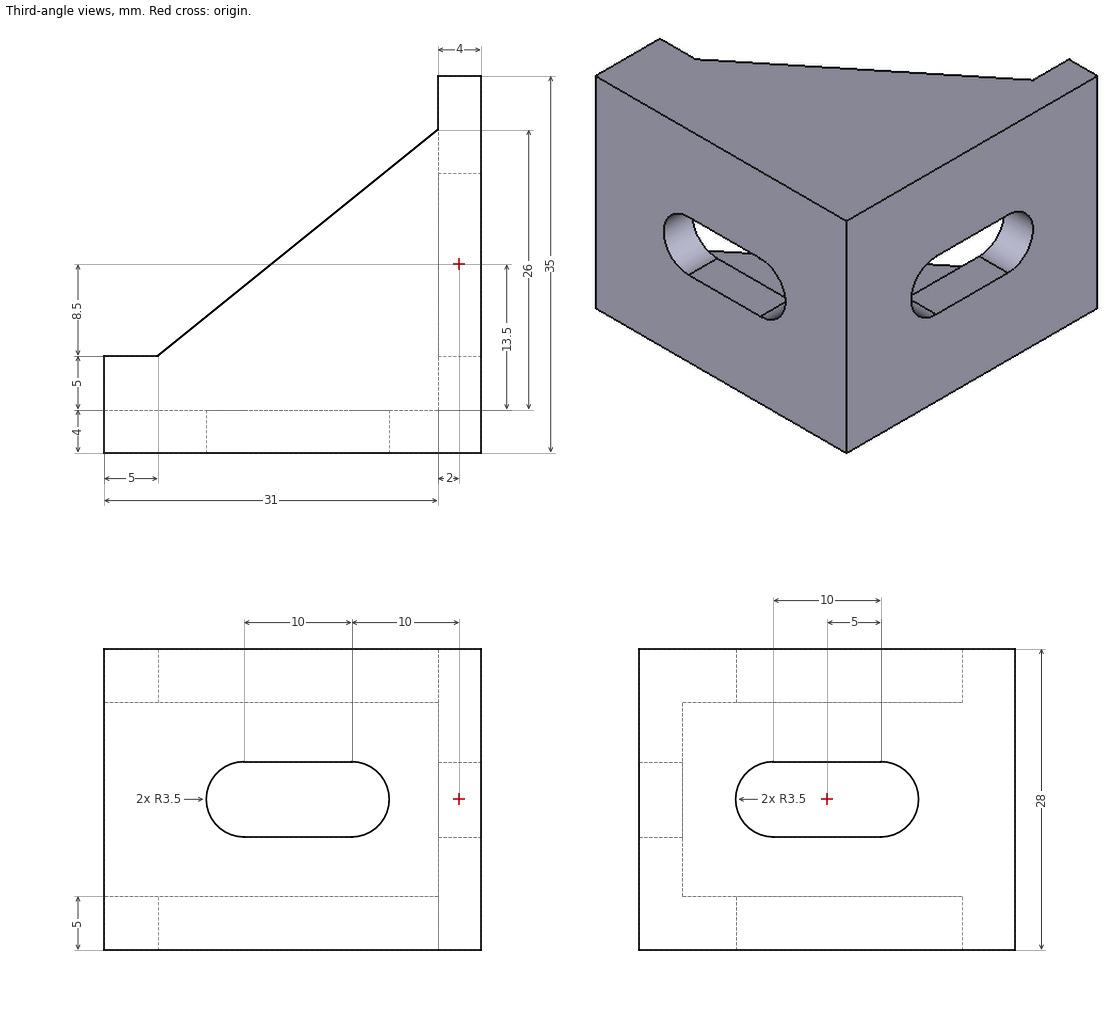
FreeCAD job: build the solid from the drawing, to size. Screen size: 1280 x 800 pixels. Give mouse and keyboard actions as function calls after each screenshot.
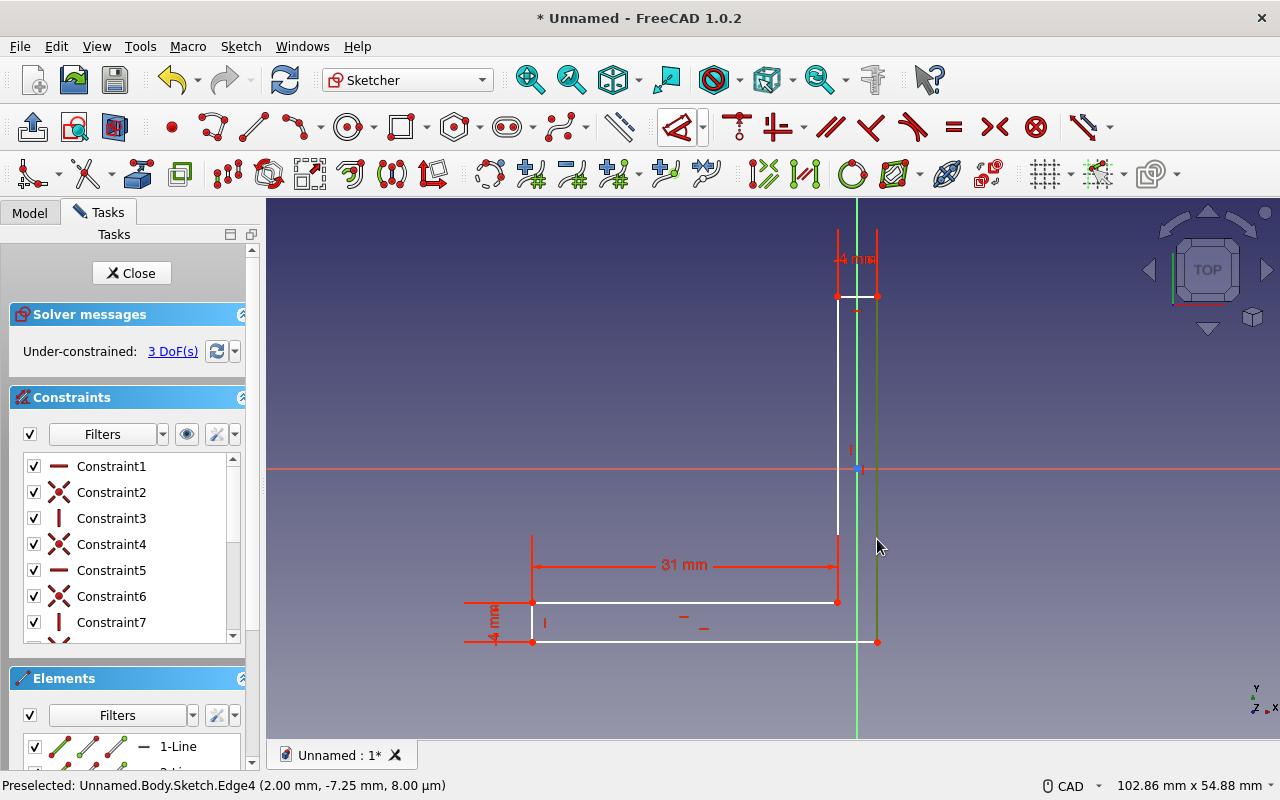
click(702, 128)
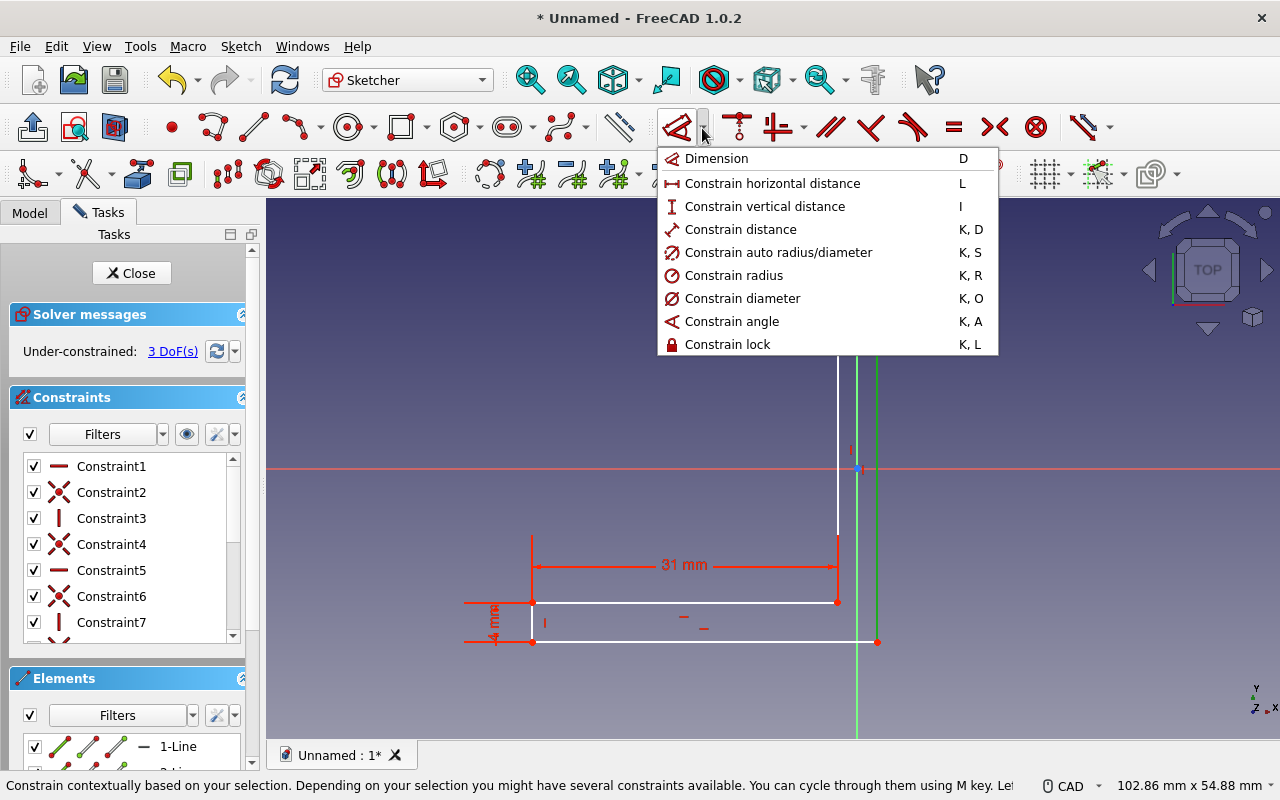
click(828, 206)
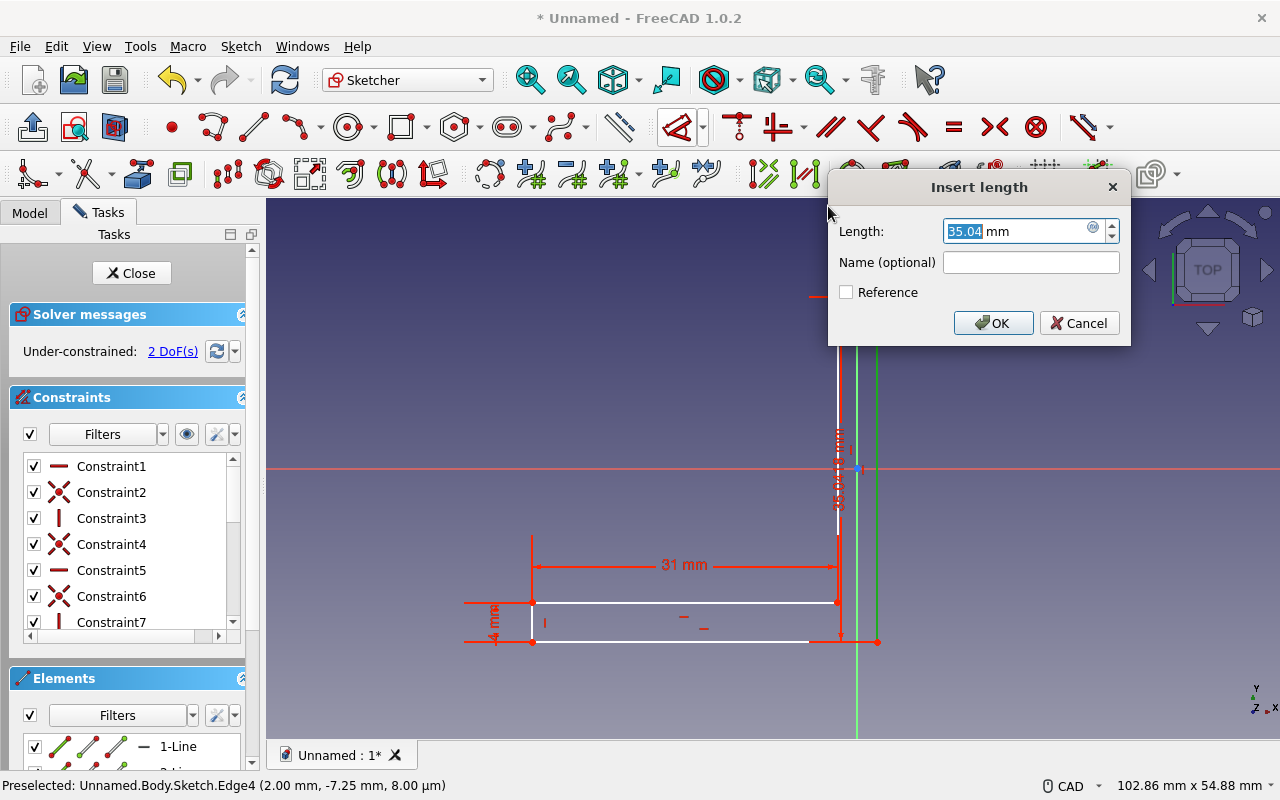
text(35)
key(Return)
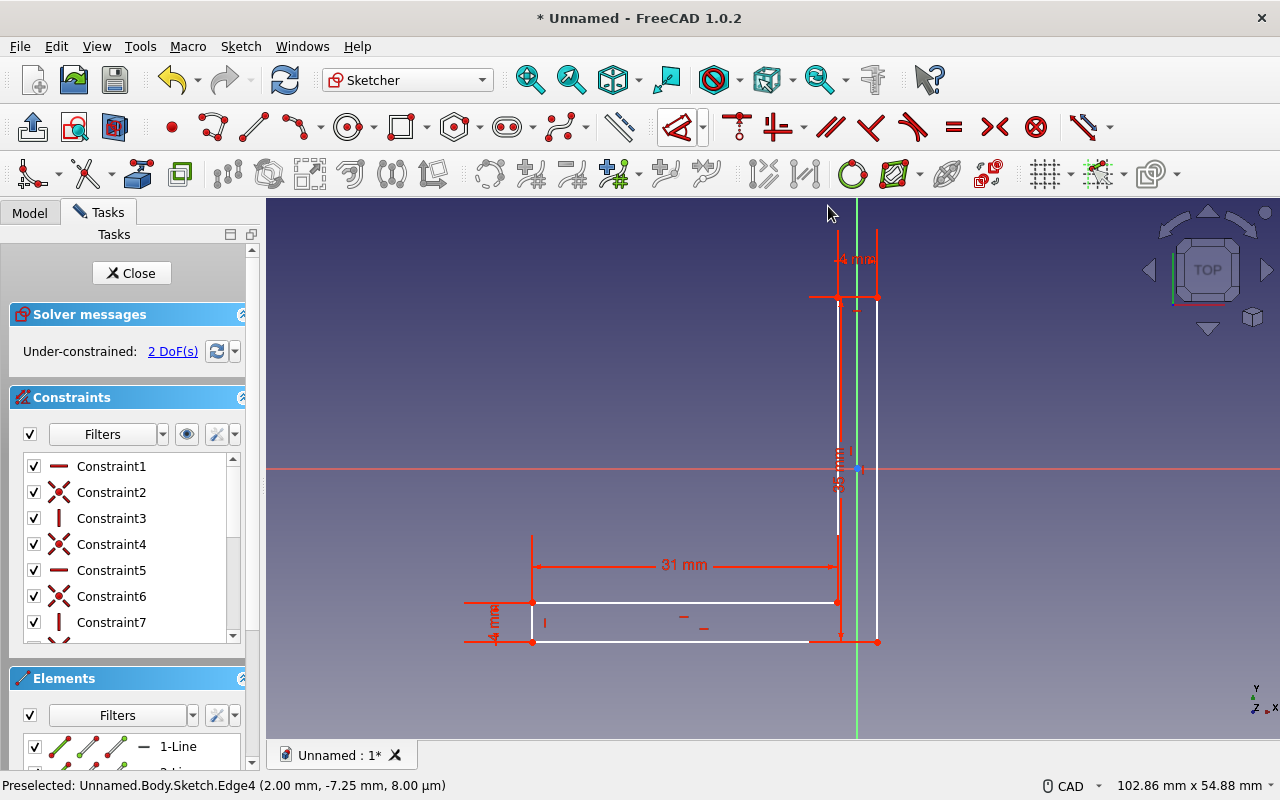
scroll(838, 603, up, 4)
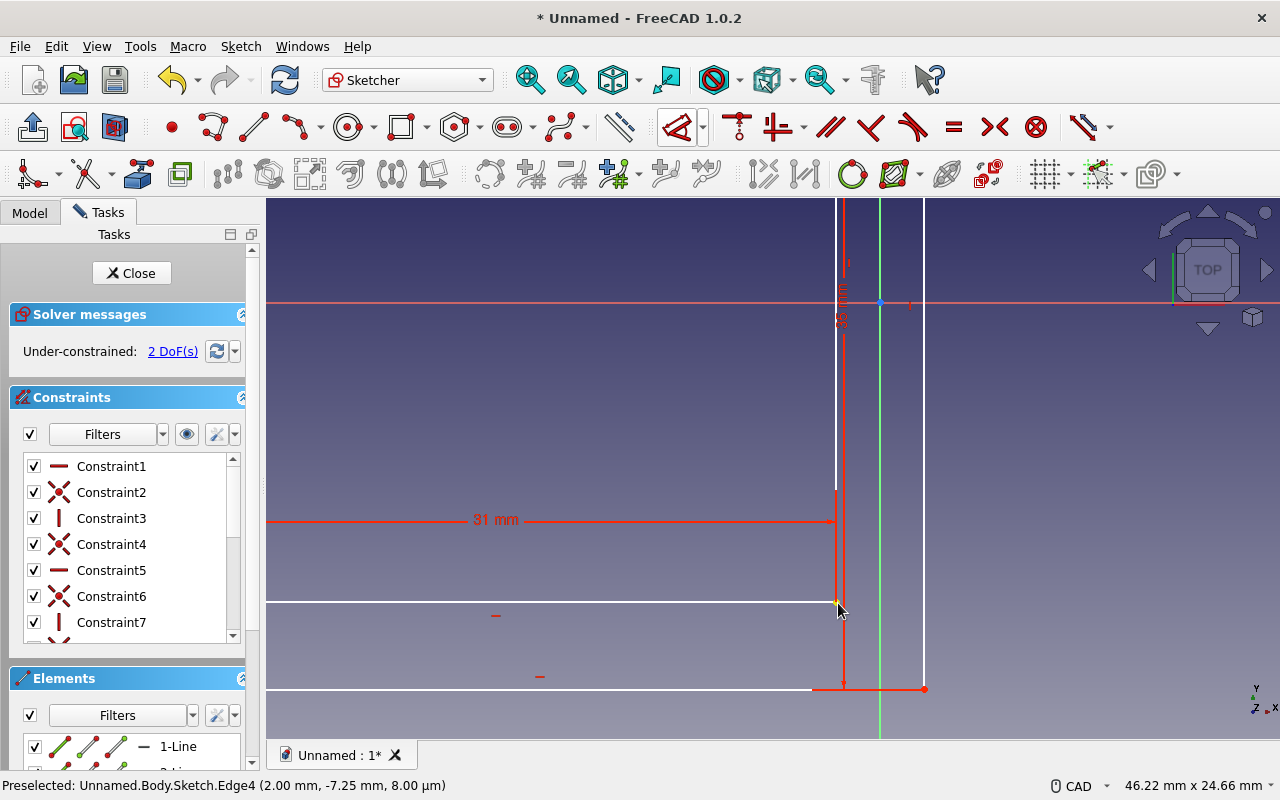
click(836, 602)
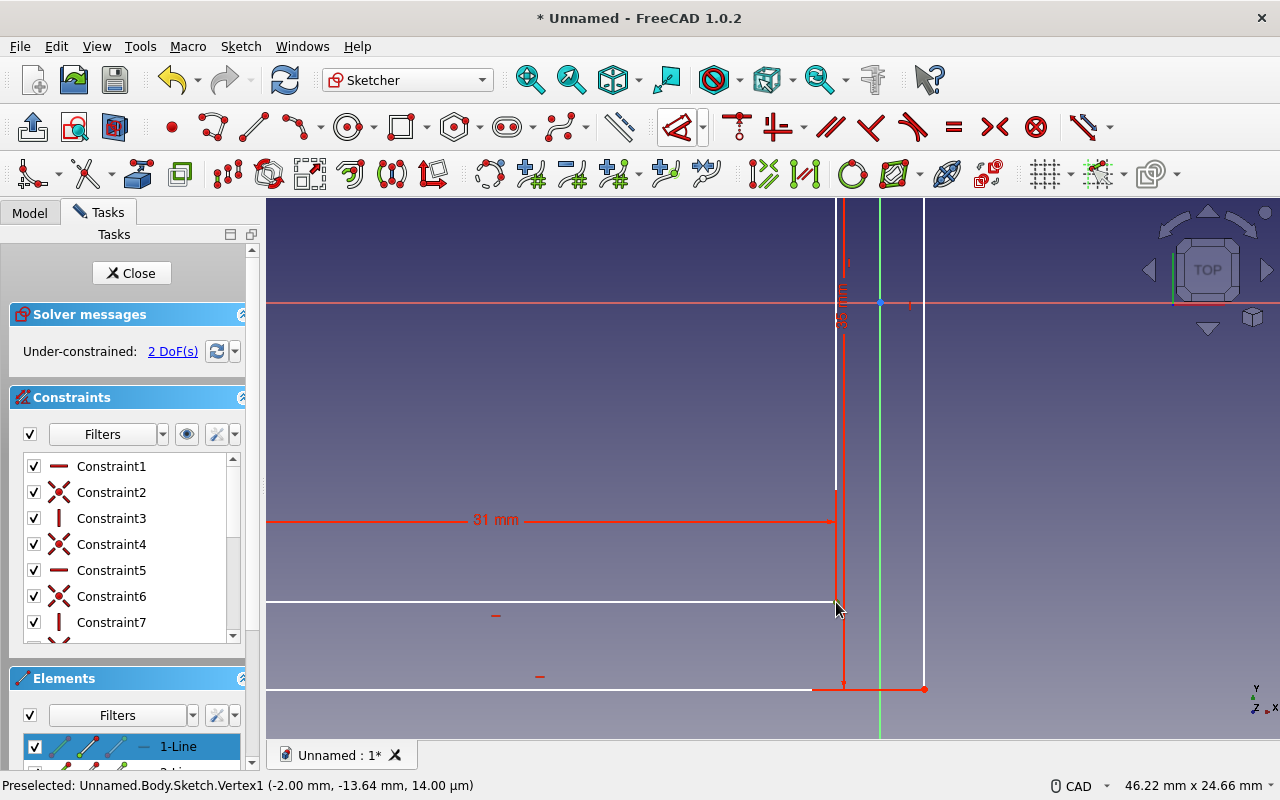
key(l)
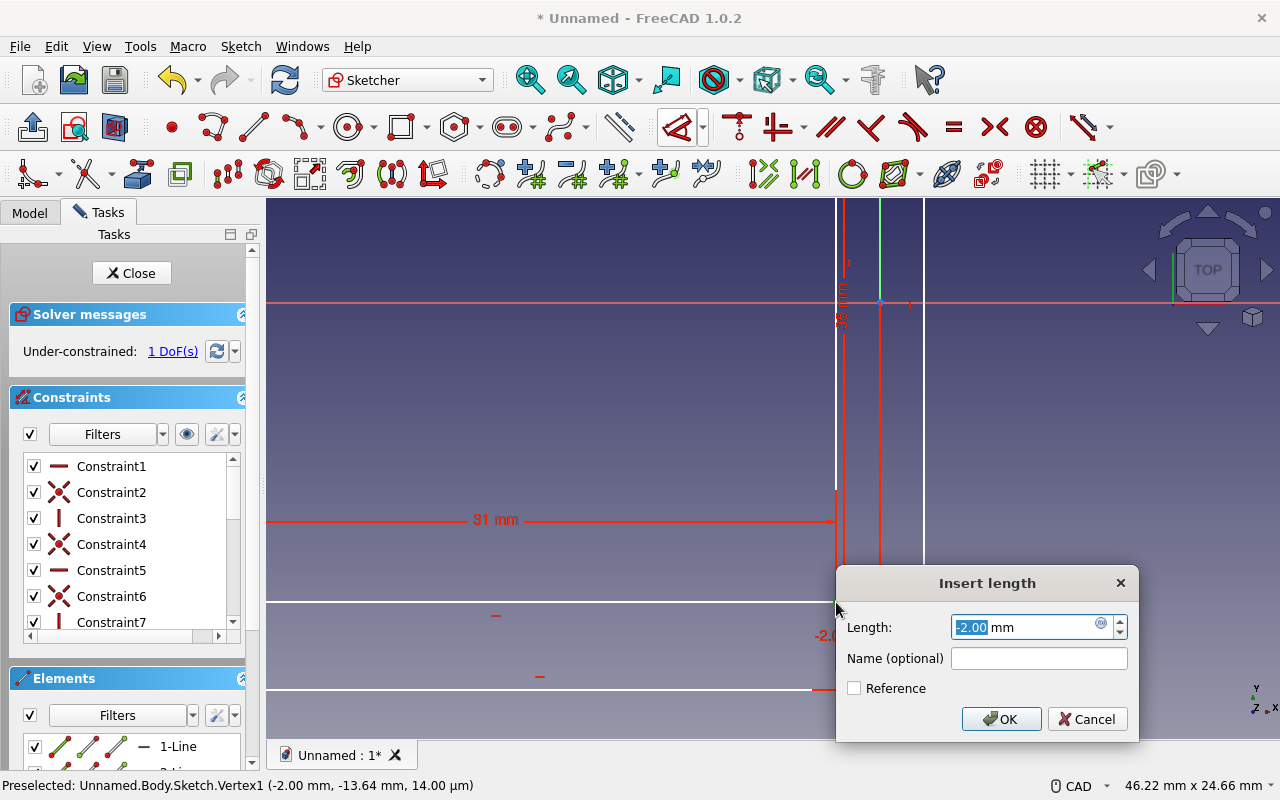
text(-2)
key(Return)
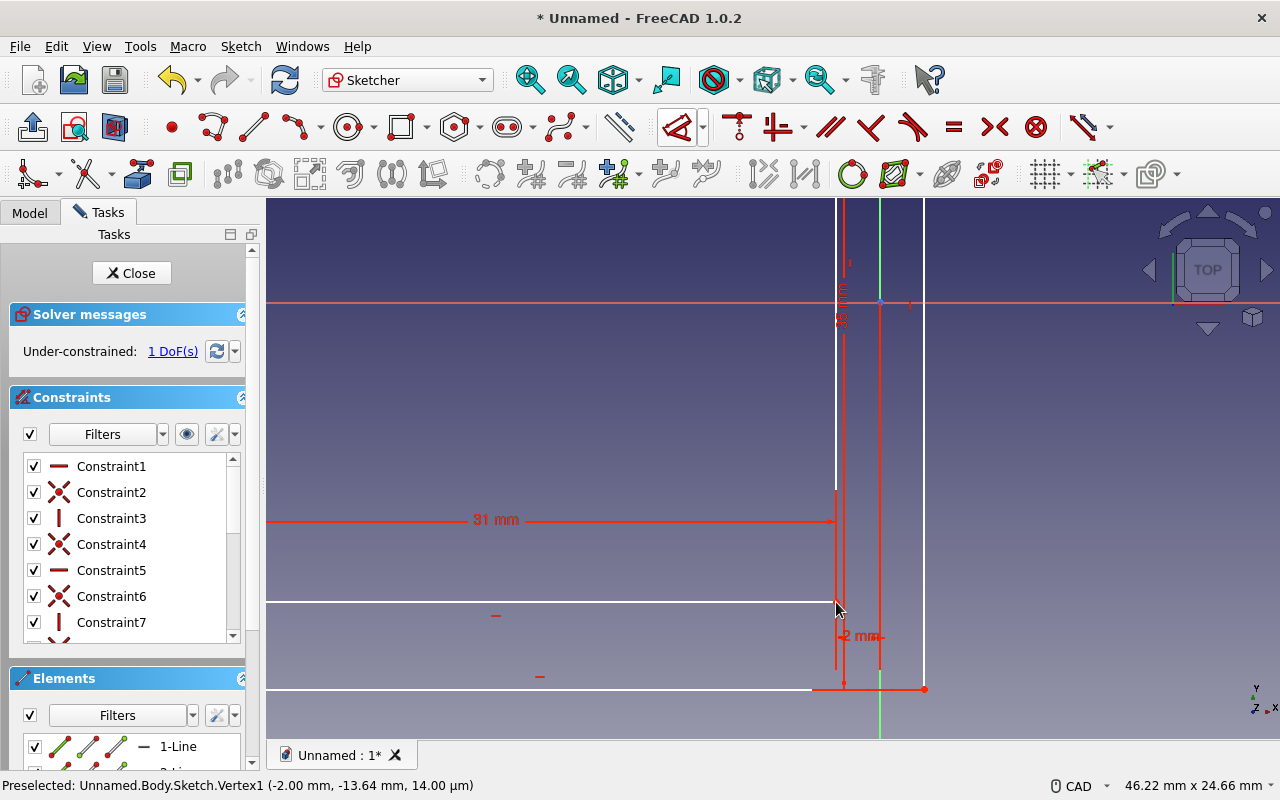
click(836, 602)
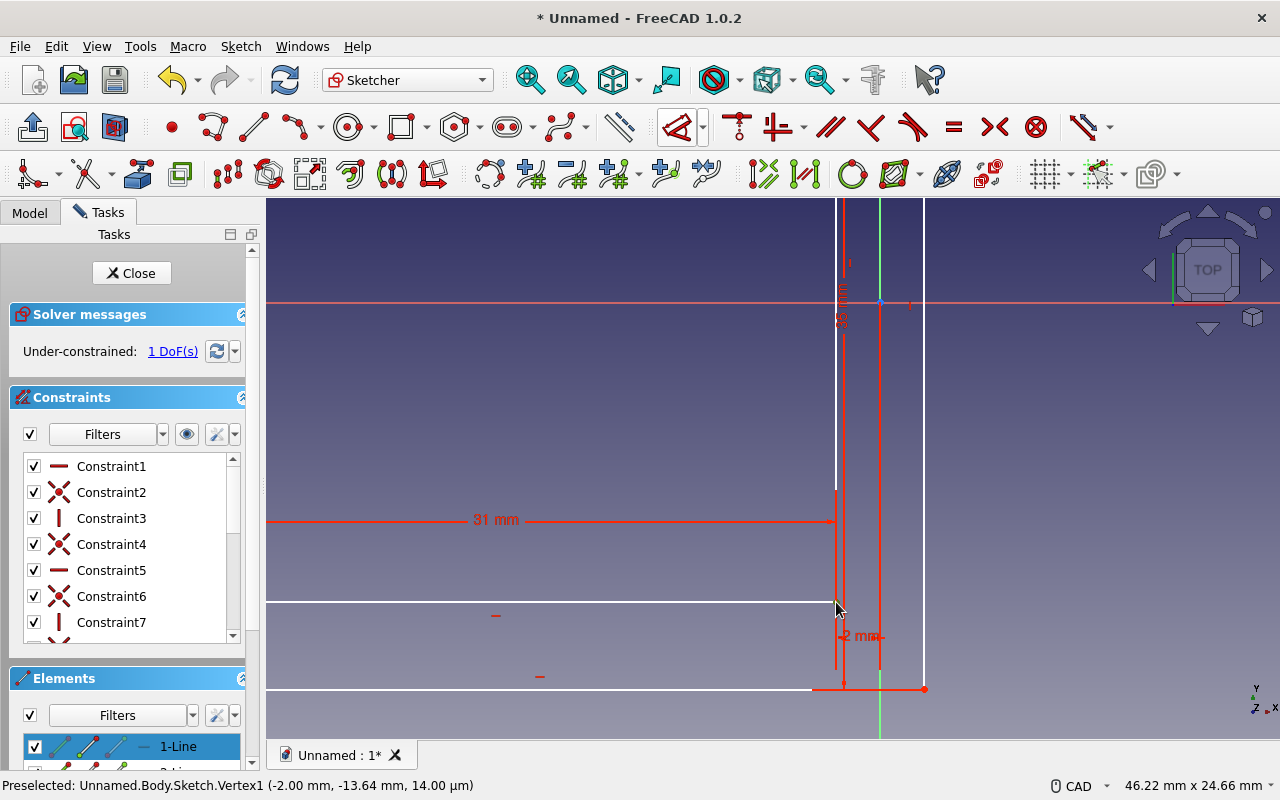
click(702, 128)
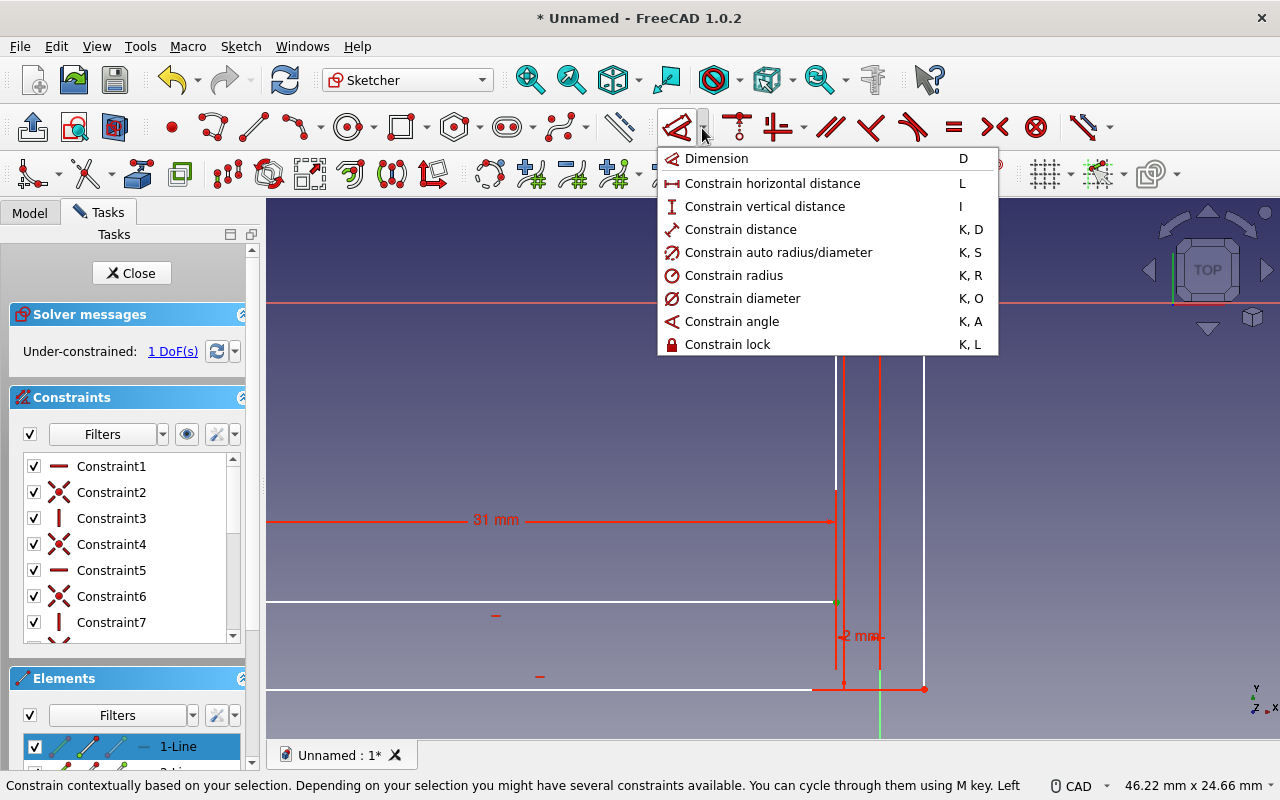
click(828, 206)